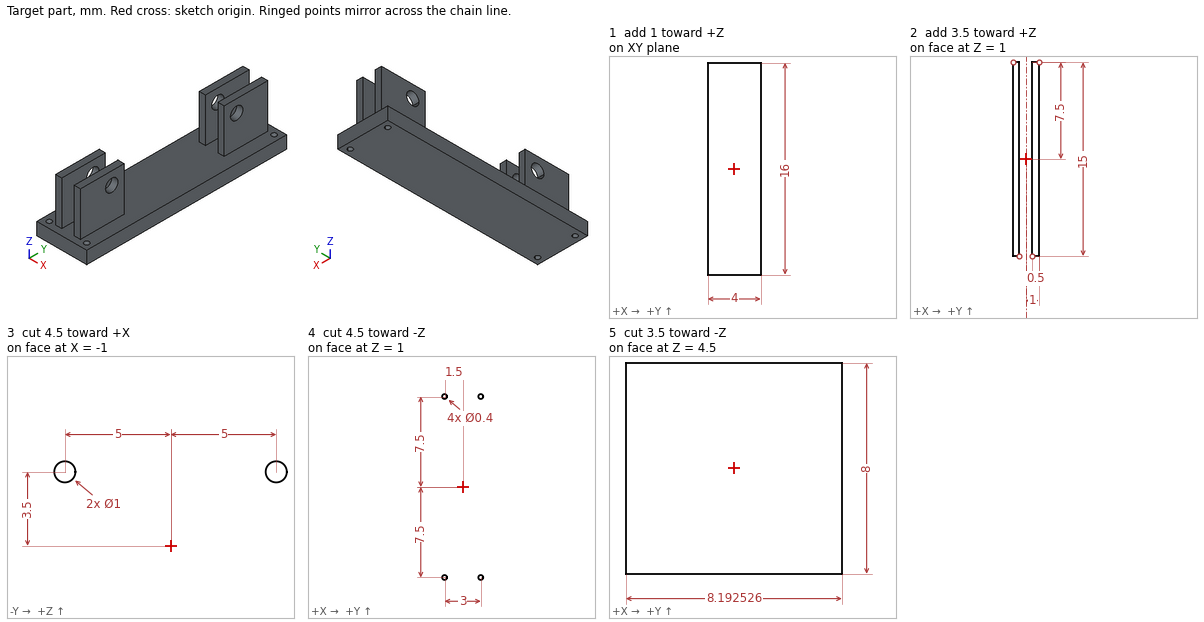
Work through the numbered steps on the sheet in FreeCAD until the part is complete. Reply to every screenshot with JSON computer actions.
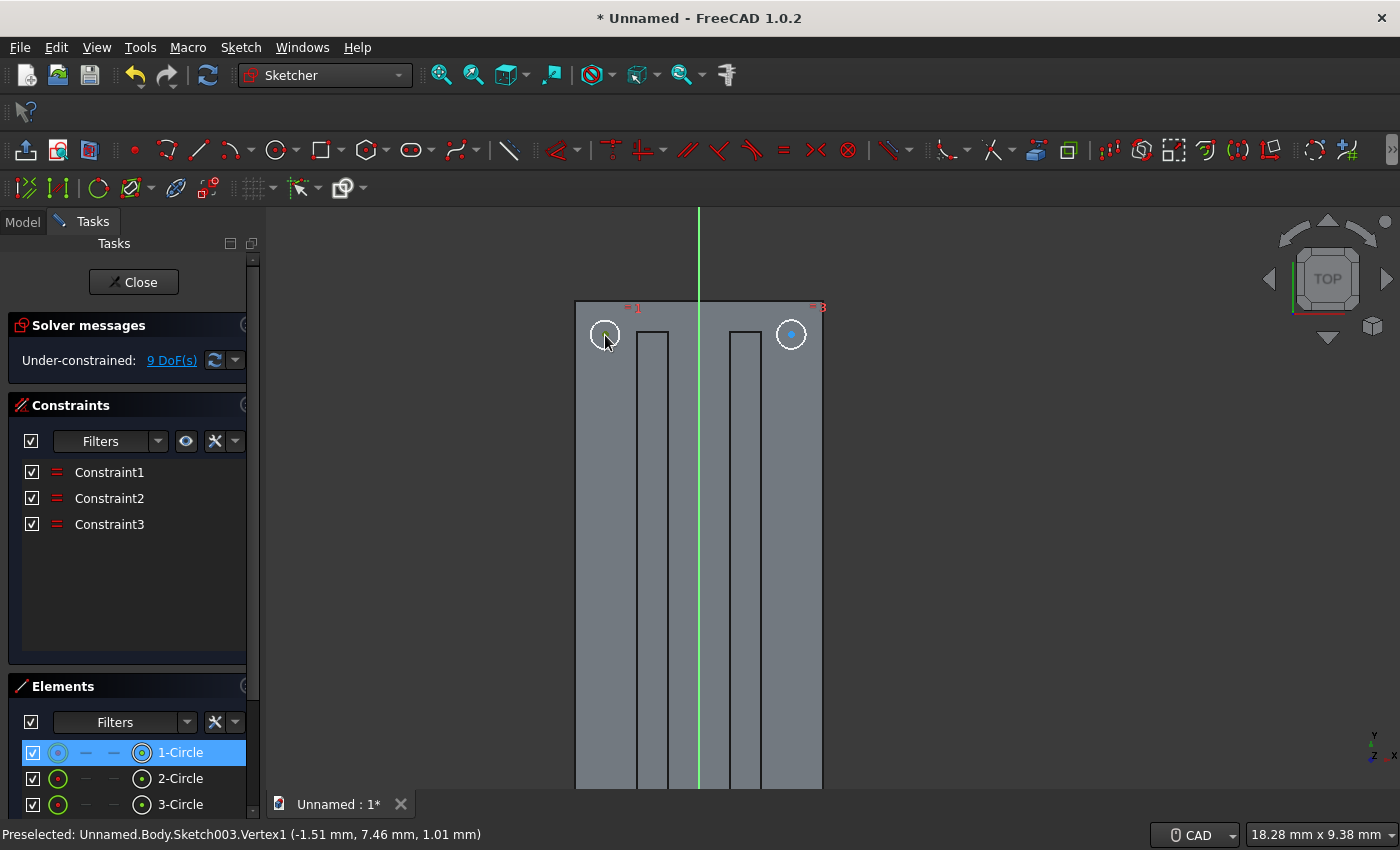
{"action": "scroll", "coordinate": [803, 324], "scroll_direction": "down", "scroll_amount": 5}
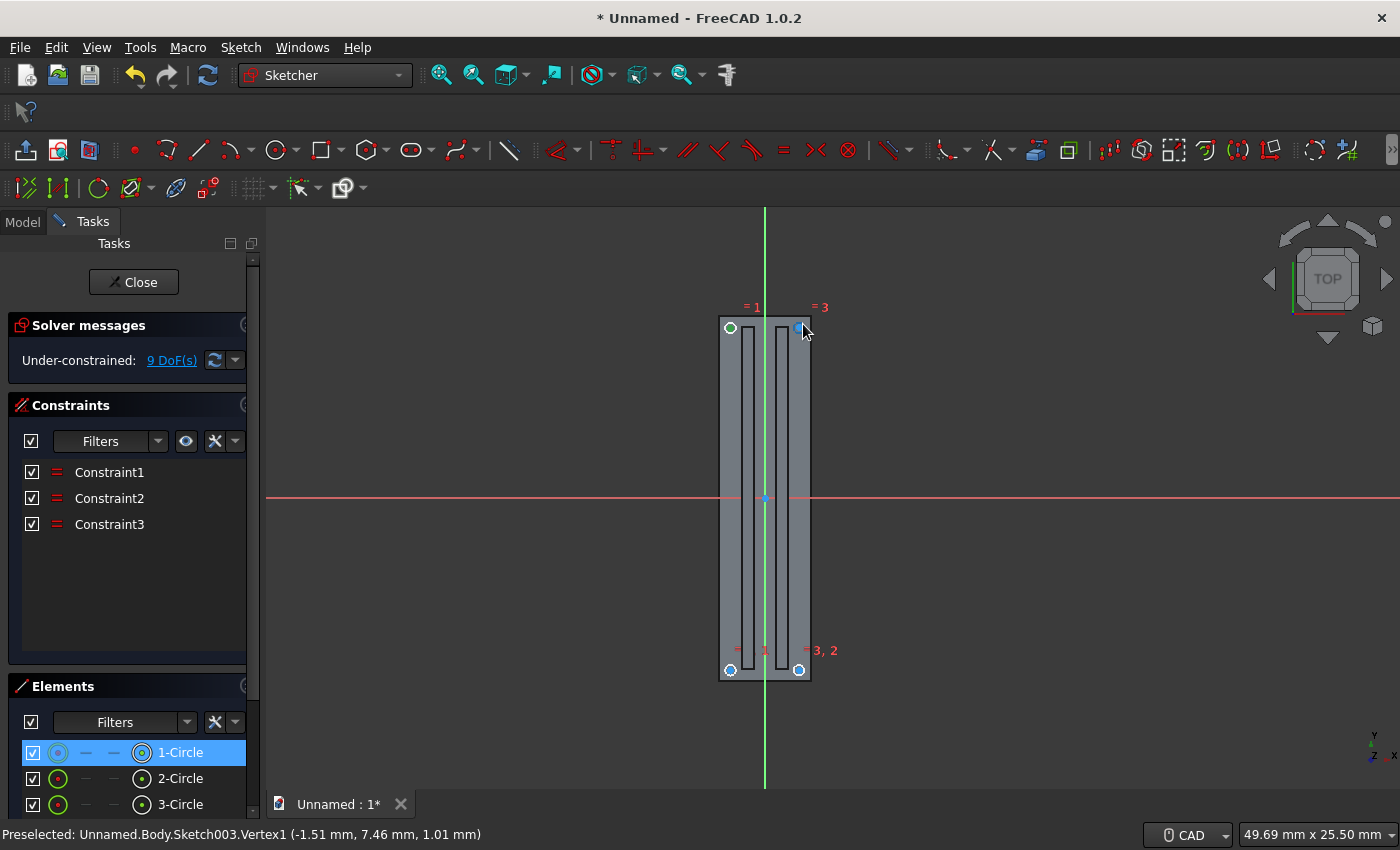
{"action": "left_click", "coordinate": [730, 670]}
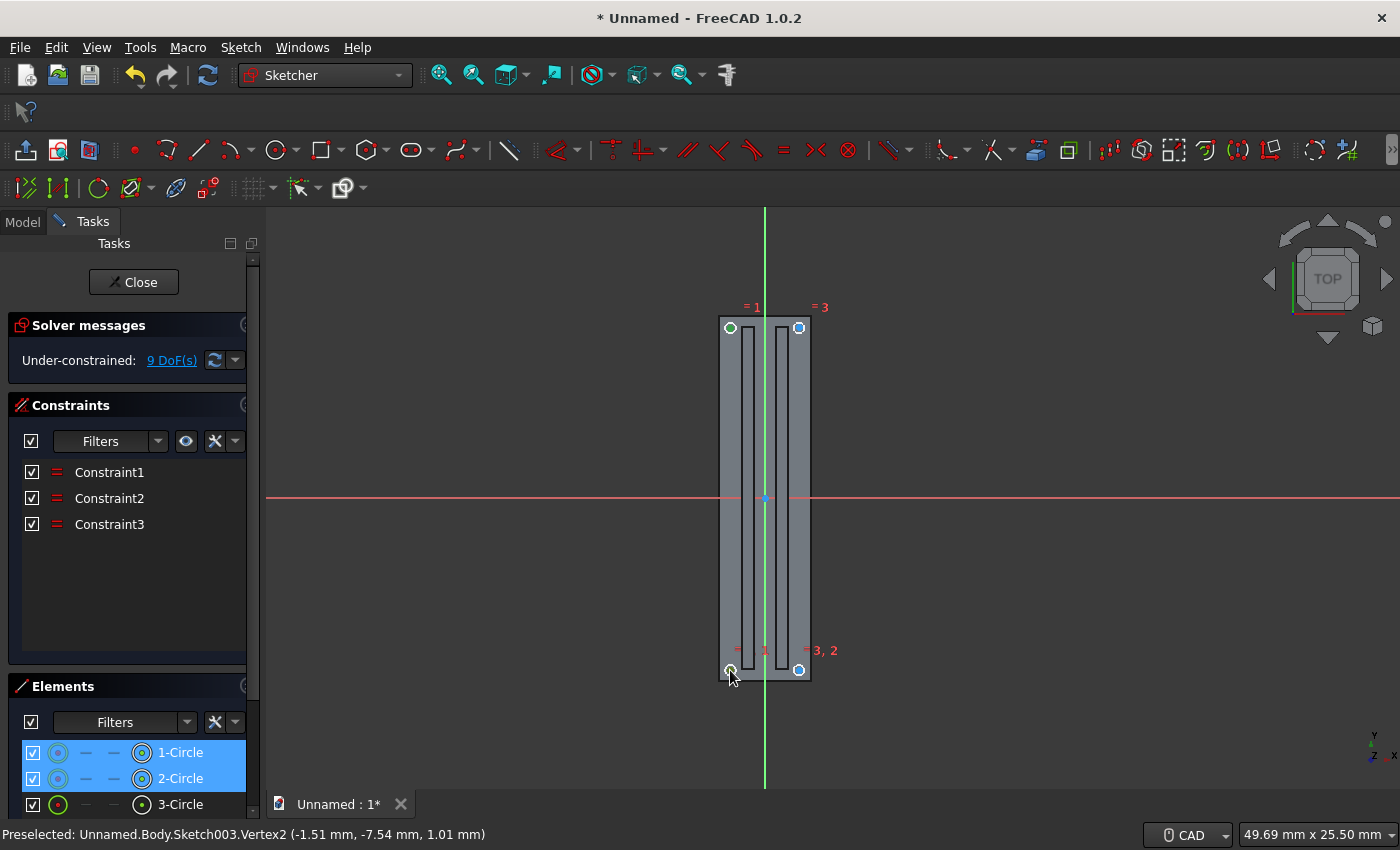
{"action": "key", "text": "v"}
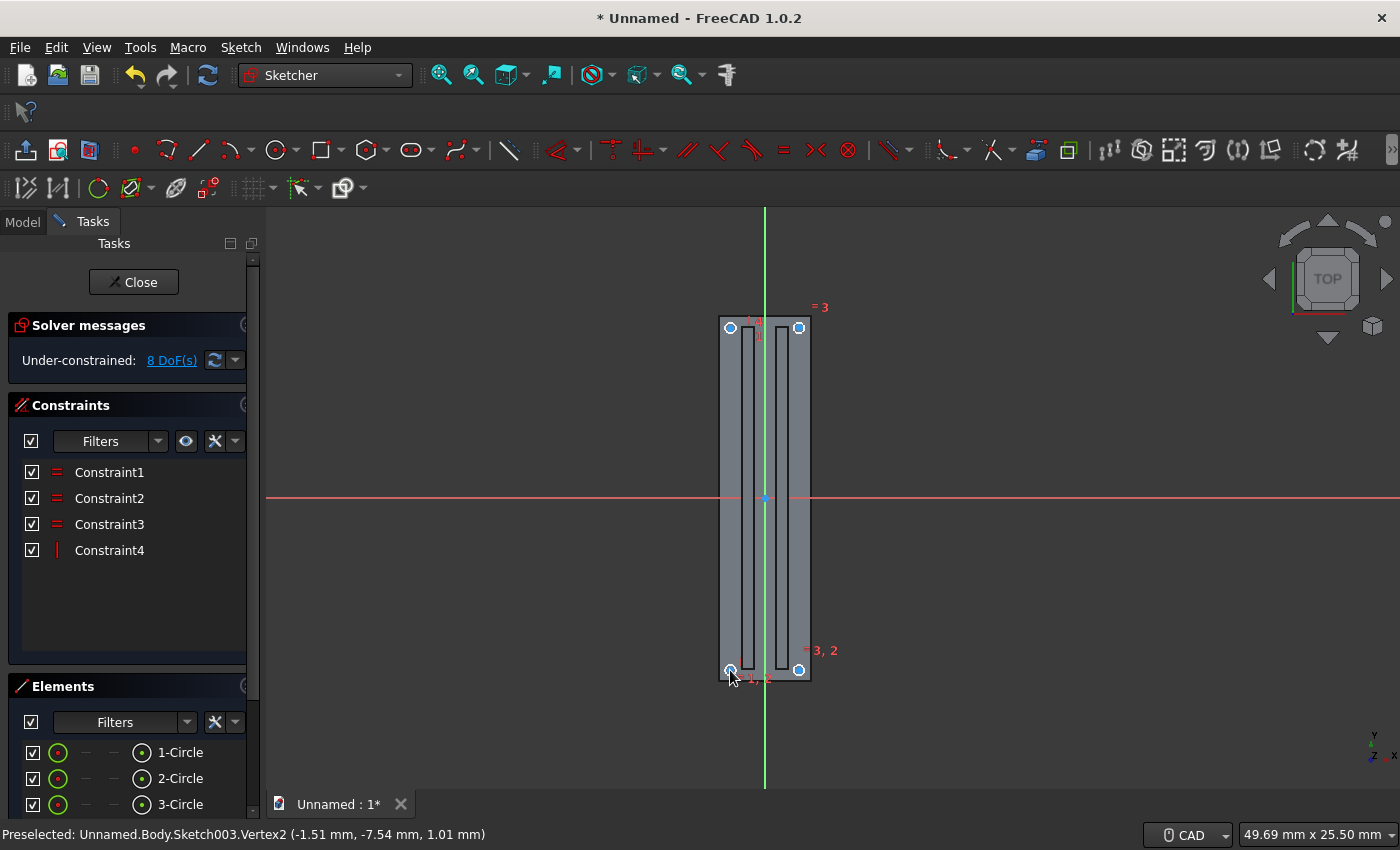
{"action": "left_click", "coordinate": [730, 670]}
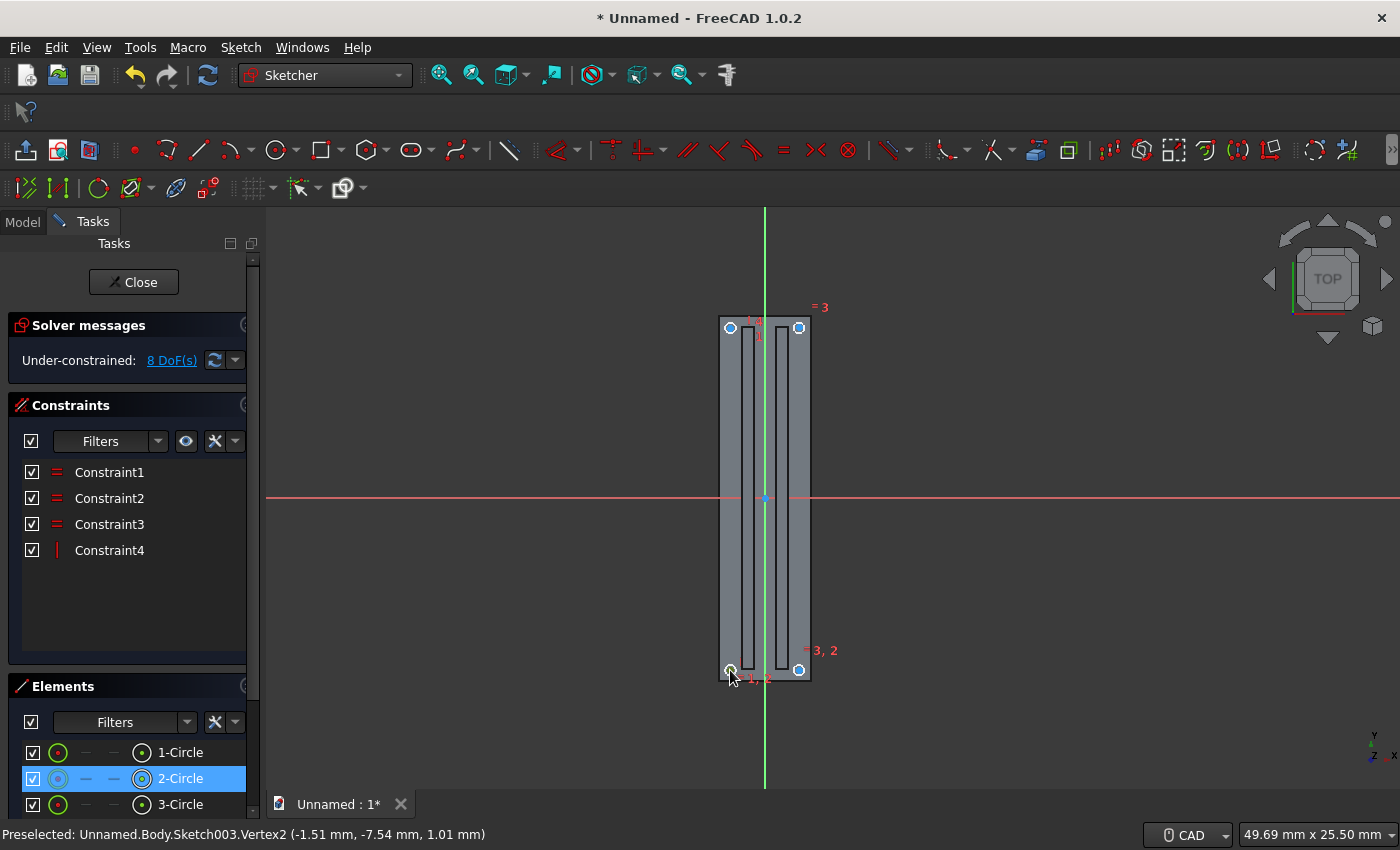
{"action": "left_click", "coordinate": [799, 670]}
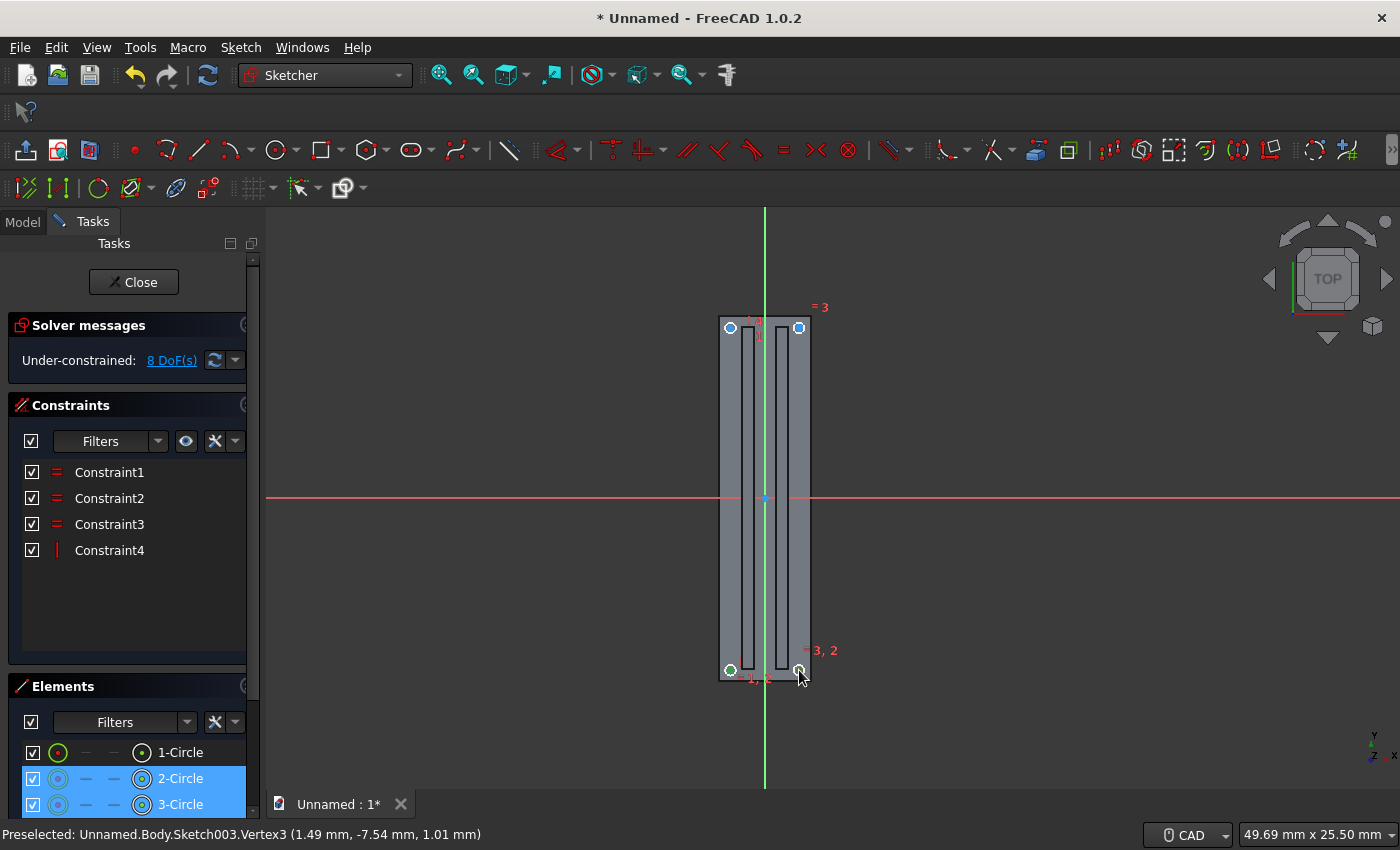
{"action": "key", "text": "h"}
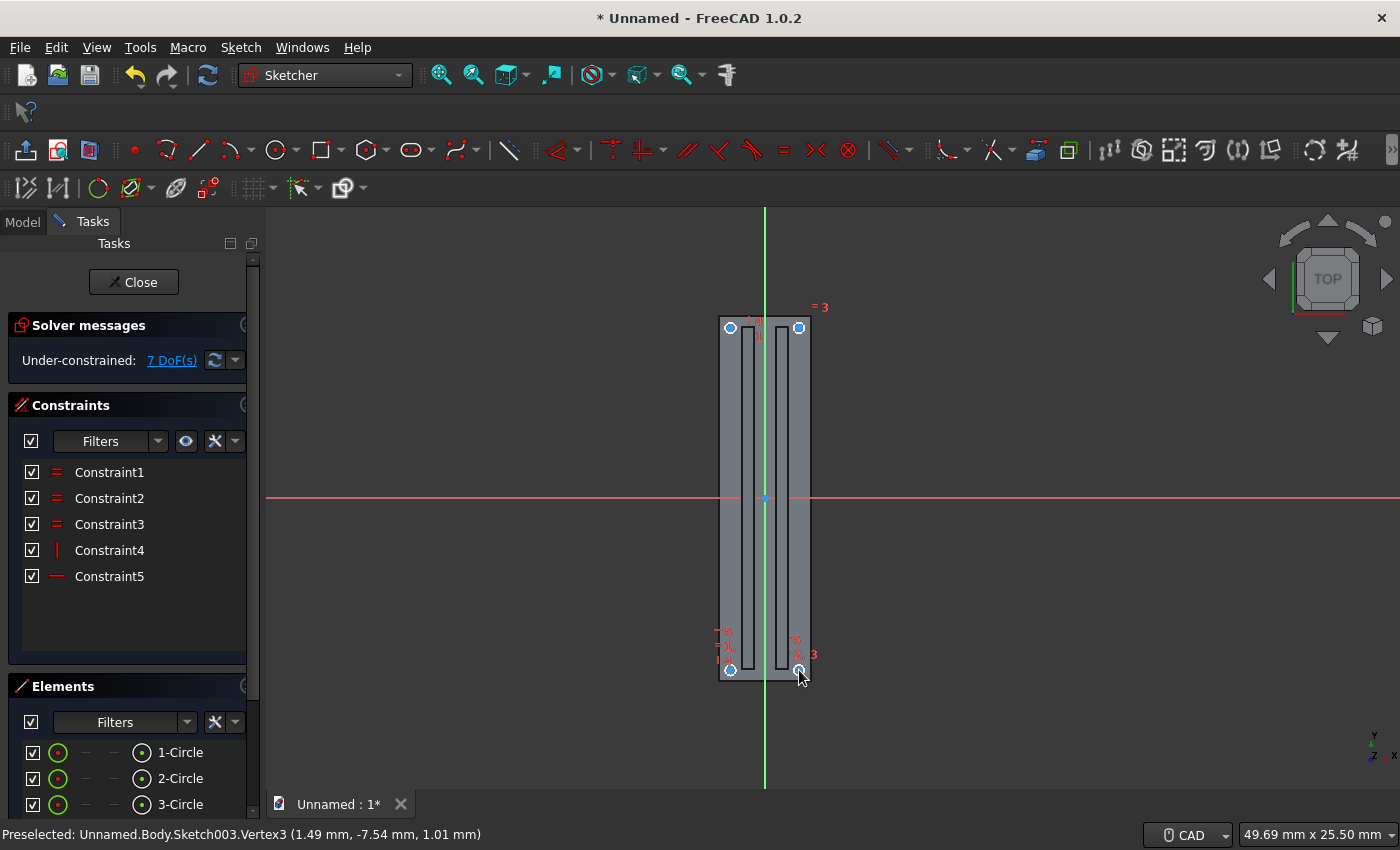
{"action": "left_click", "coordinate": [799, 670]}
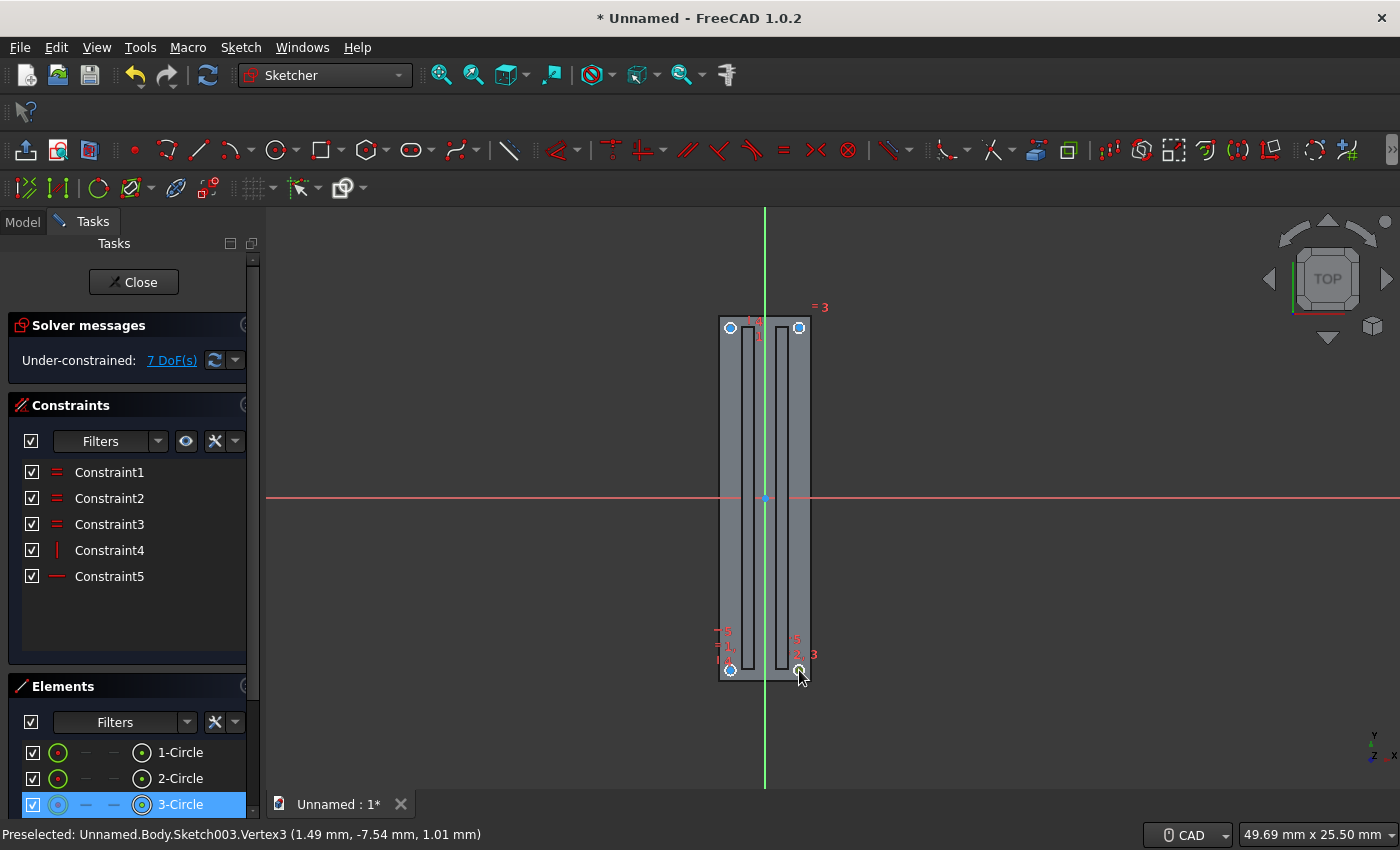
{"action": "left_click", "coordinate": [799, 328]}